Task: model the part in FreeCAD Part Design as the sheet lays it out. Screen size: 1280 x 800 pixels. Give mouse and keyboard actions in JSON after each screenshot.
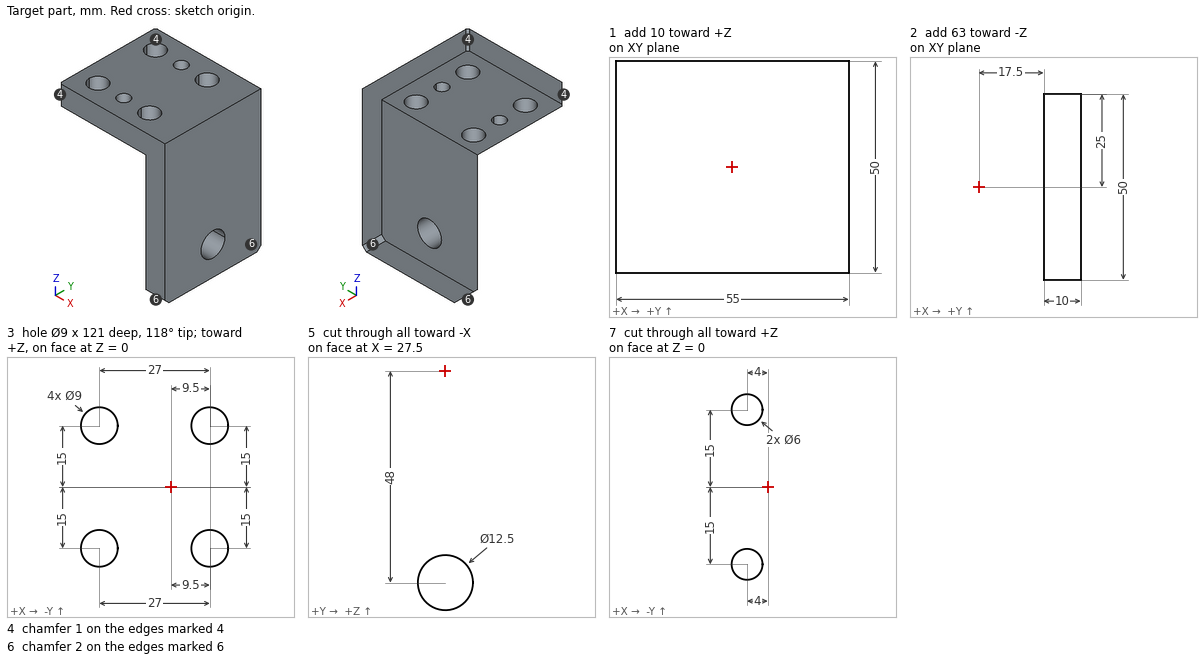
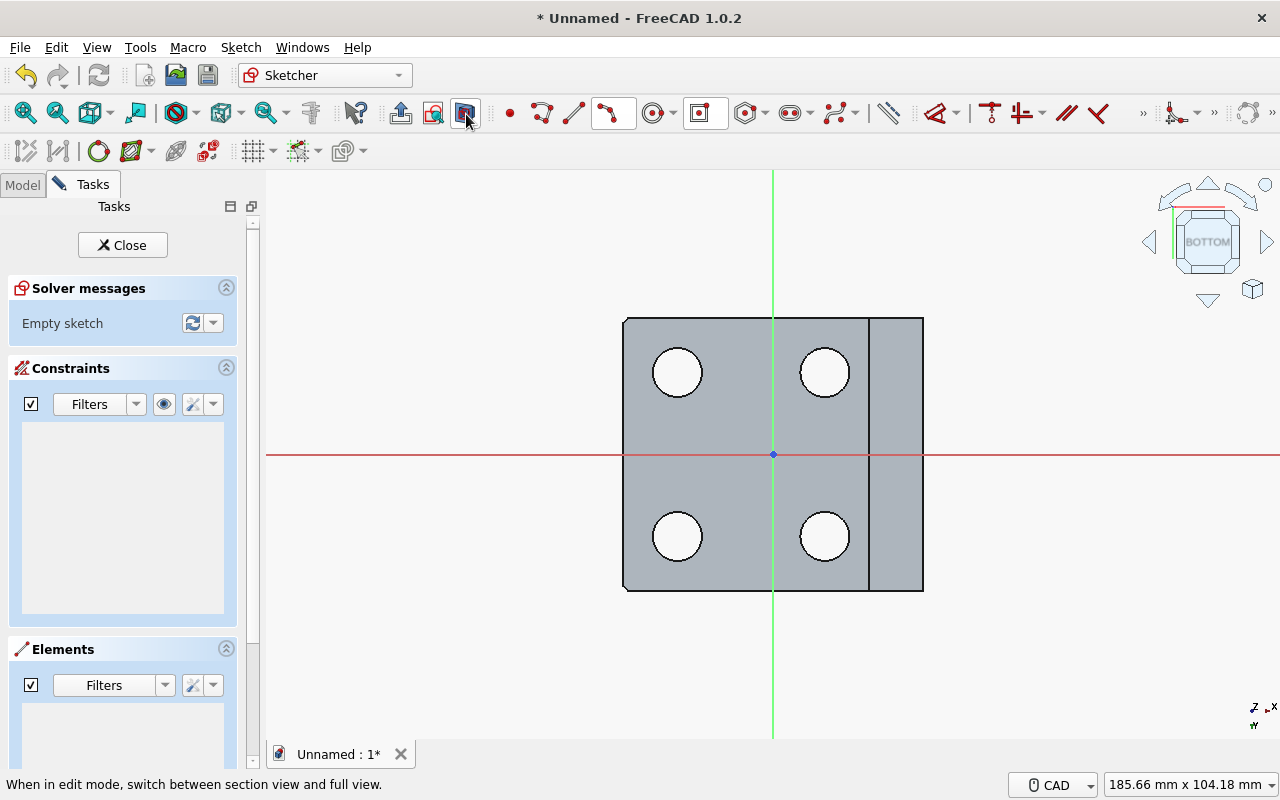
{"action": "scroll", "coordinate": [814, 455], "scroll_direction": "up", "scroll_amount": 3}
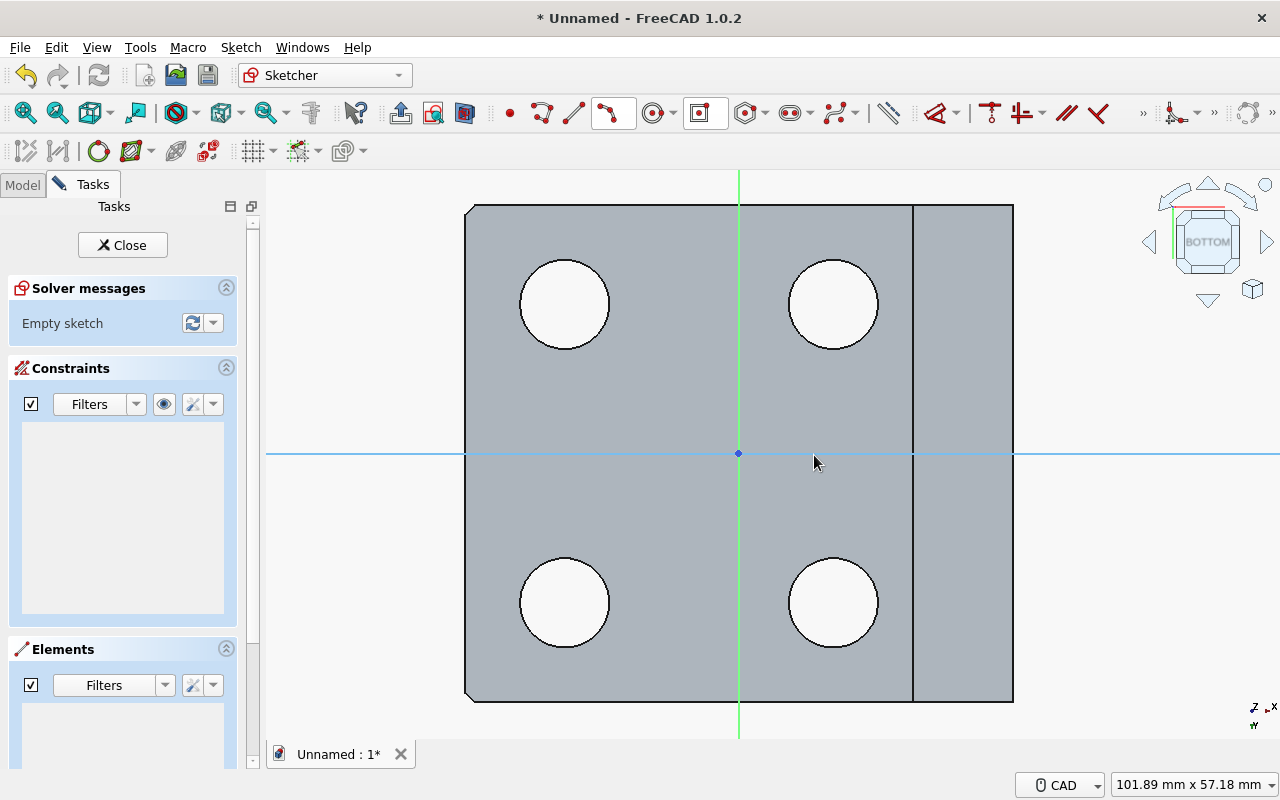
{"action": "left_click", "coordinate": [654, 114]}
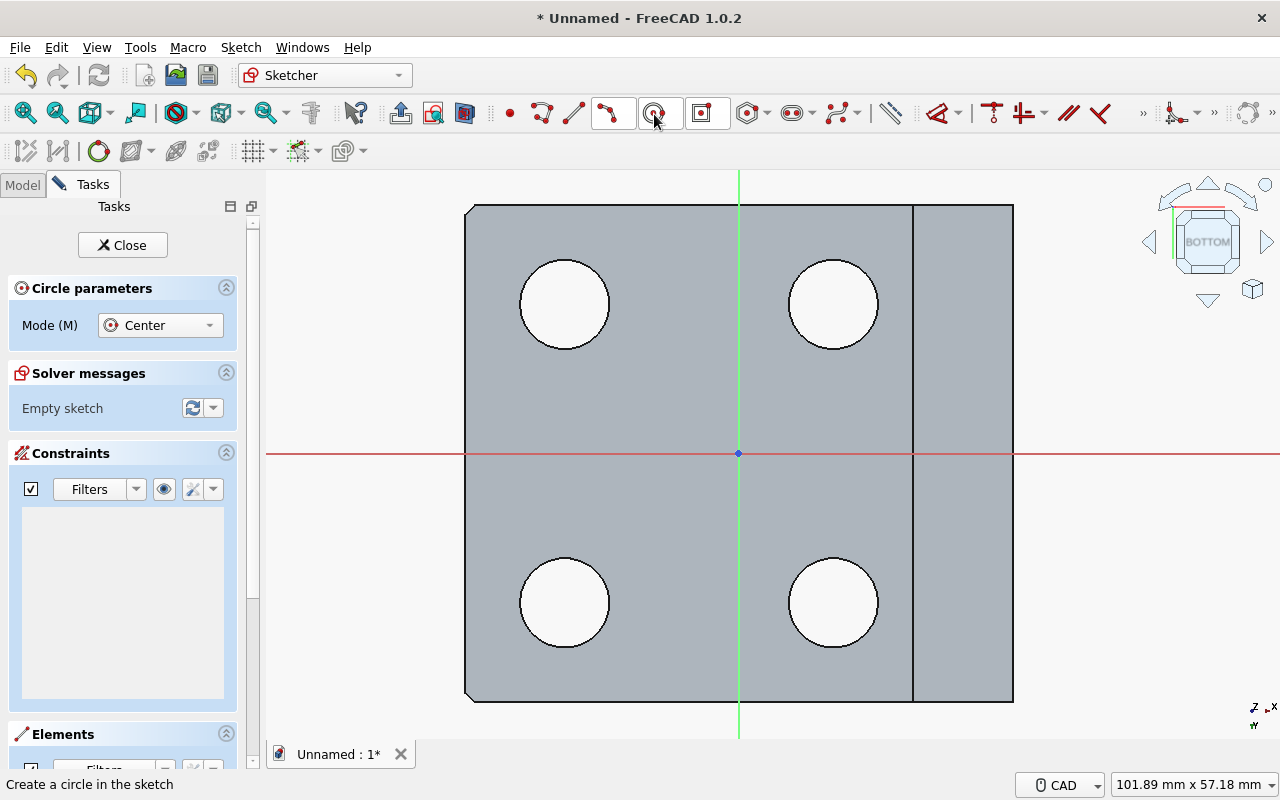
{"action": "left_click", "coordinate": [699, 304]}
{"action": "left_click", "coordinate": [720, 283]}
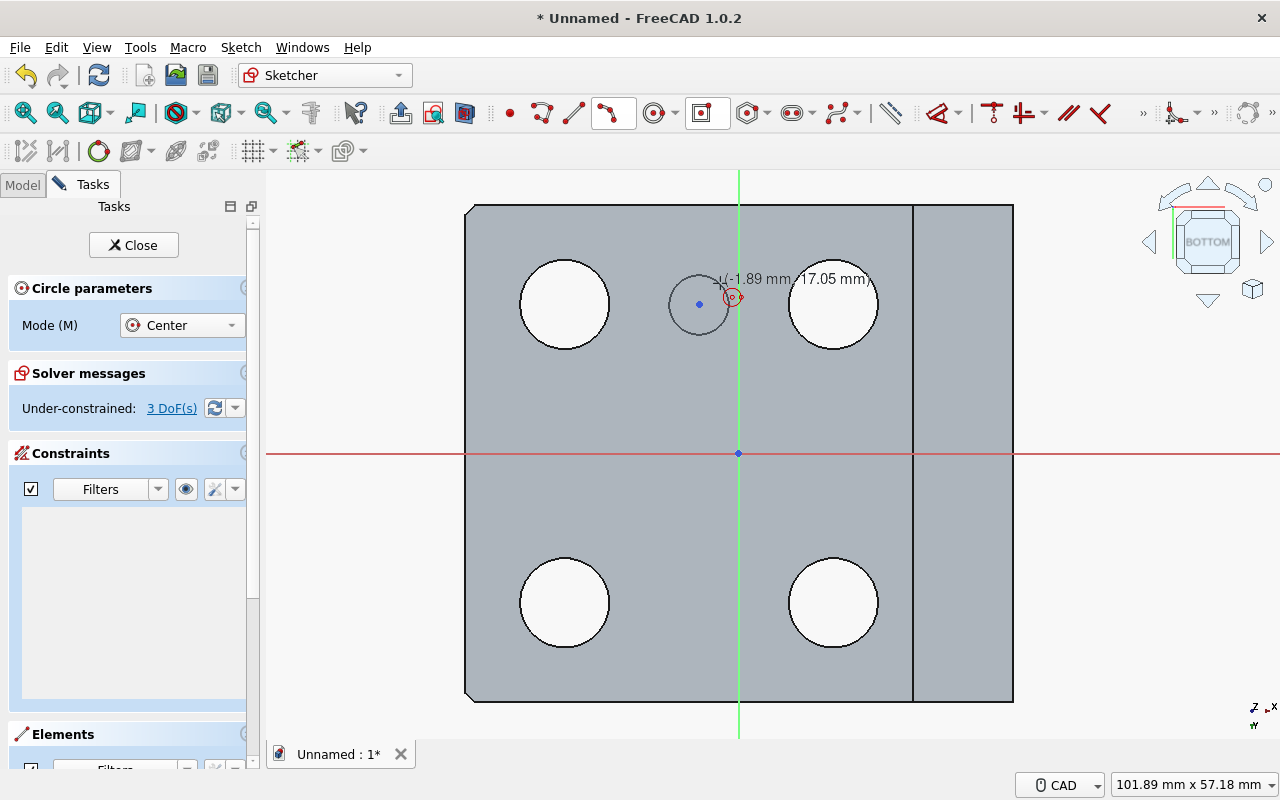
{"action": "left_click", "coordinate": [699, 603]}
{"action": "left_click", "coordinate": [720, 582]}
{"action": "key", "text": "Escape"}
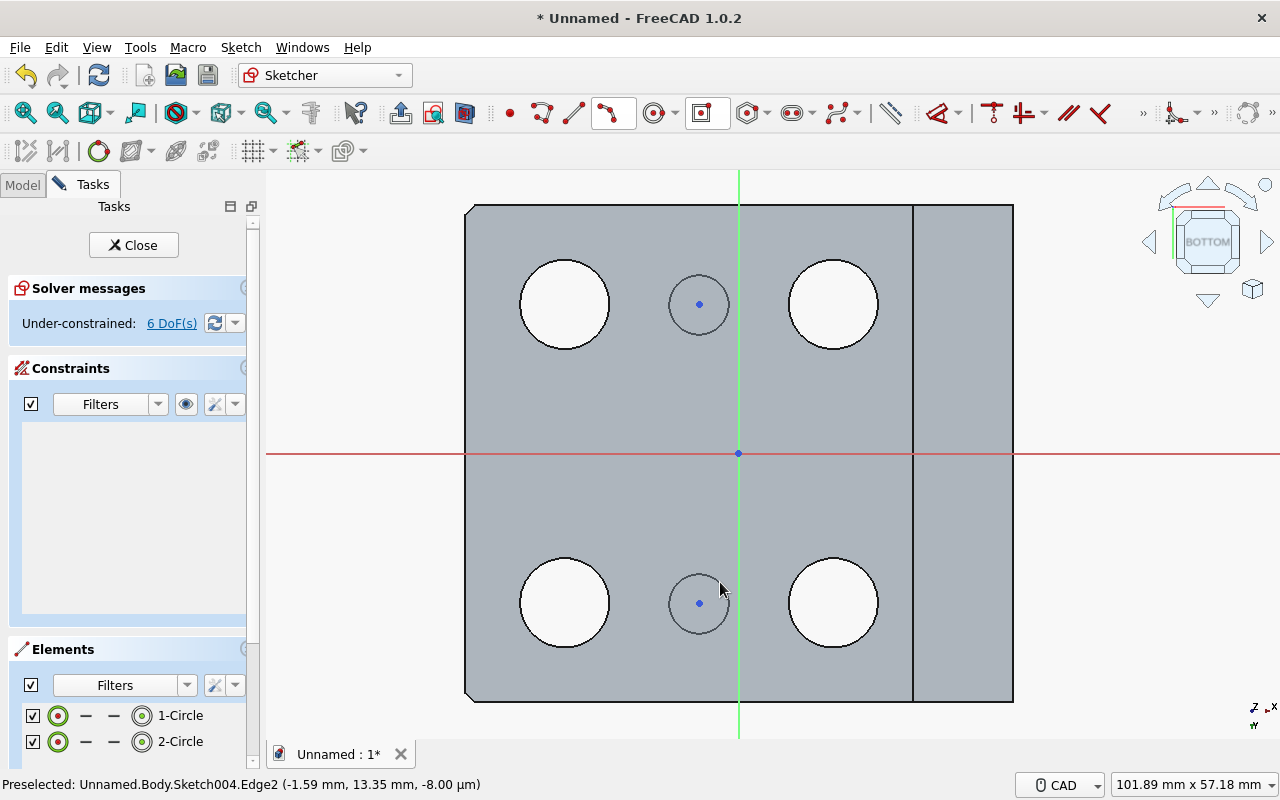
{"action": "left_click", "coordinate": [720, 284]}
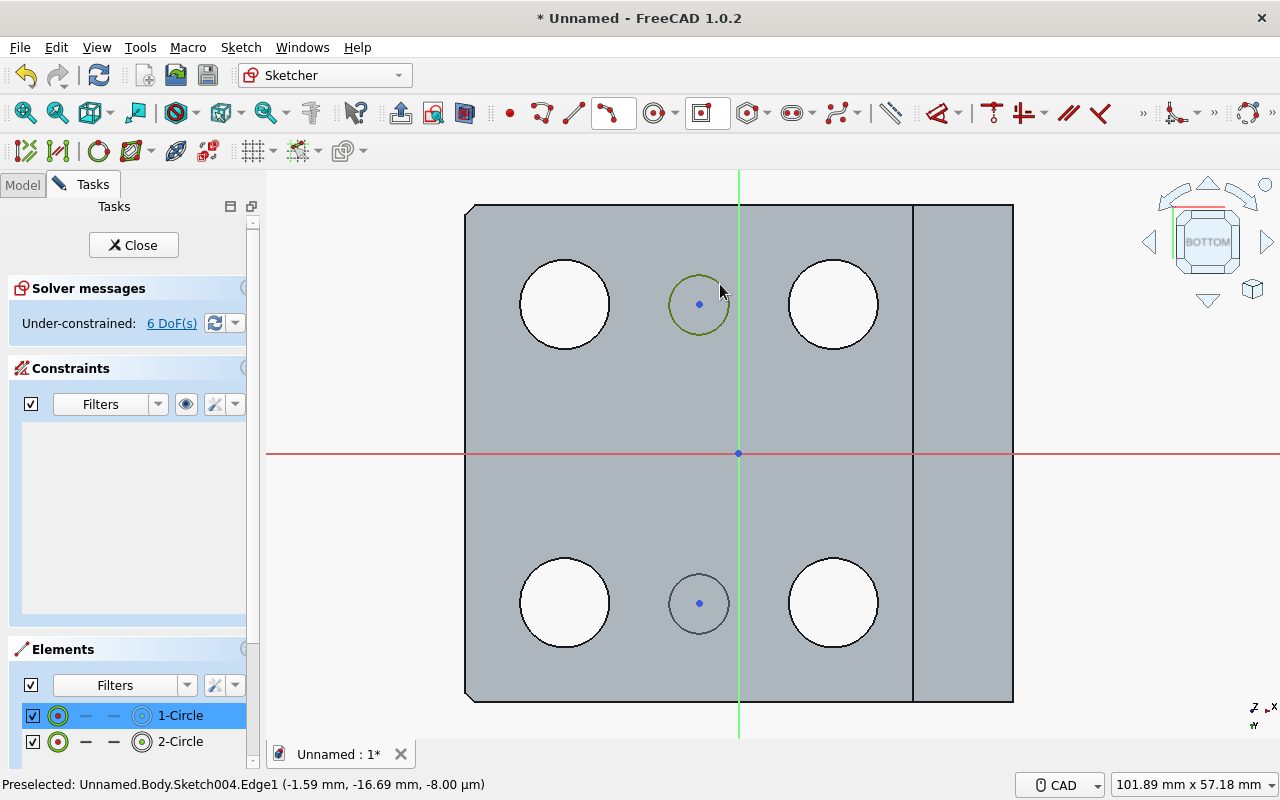
{"action": "left_click", "coordinate": [720, 583]}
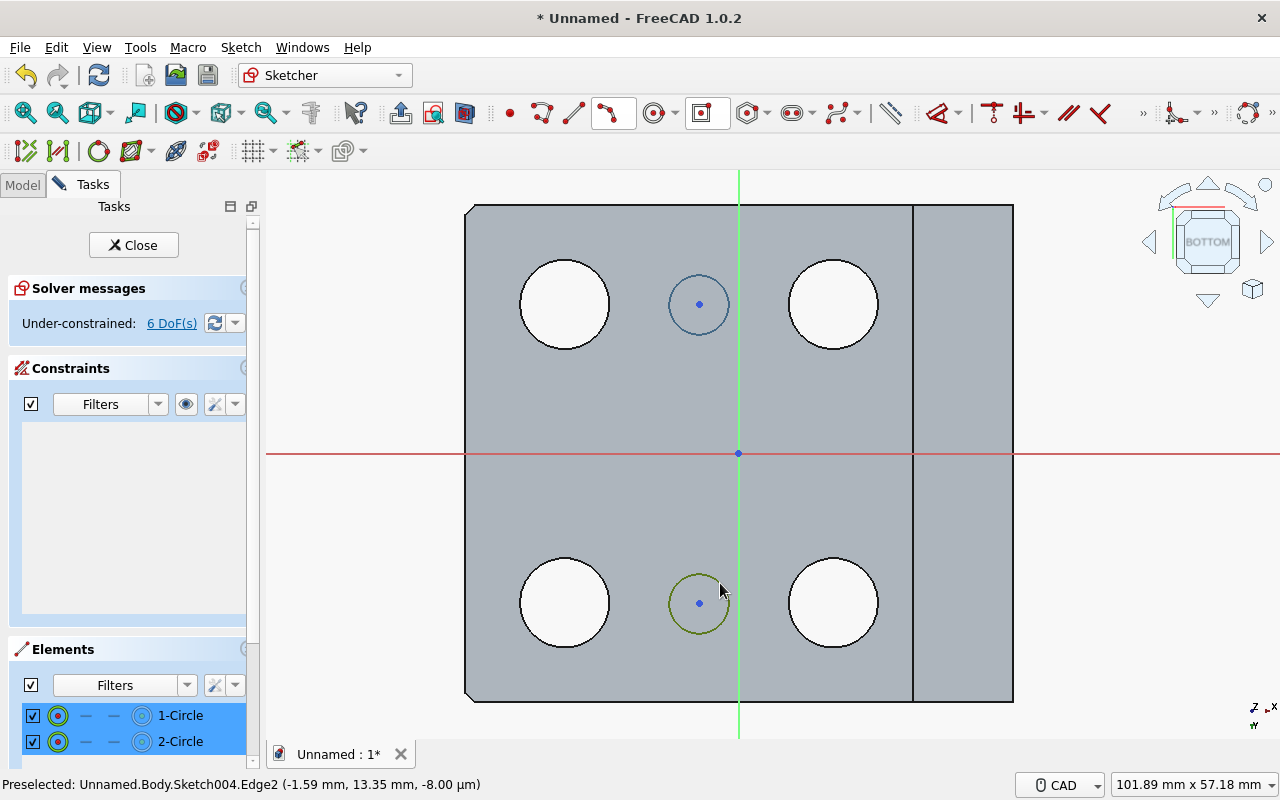
{"action": "key", "text": "e"}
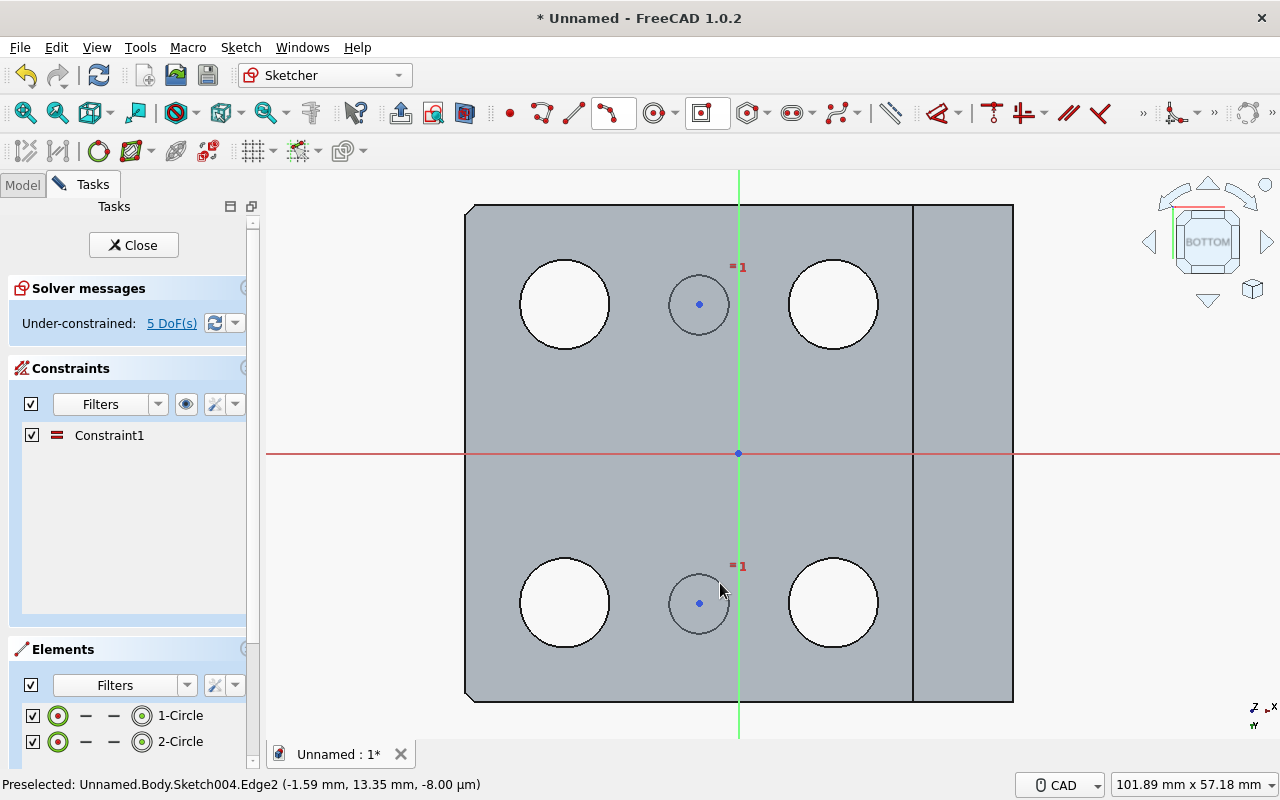
{"action": "left_click", "coordinate": [938, 114]}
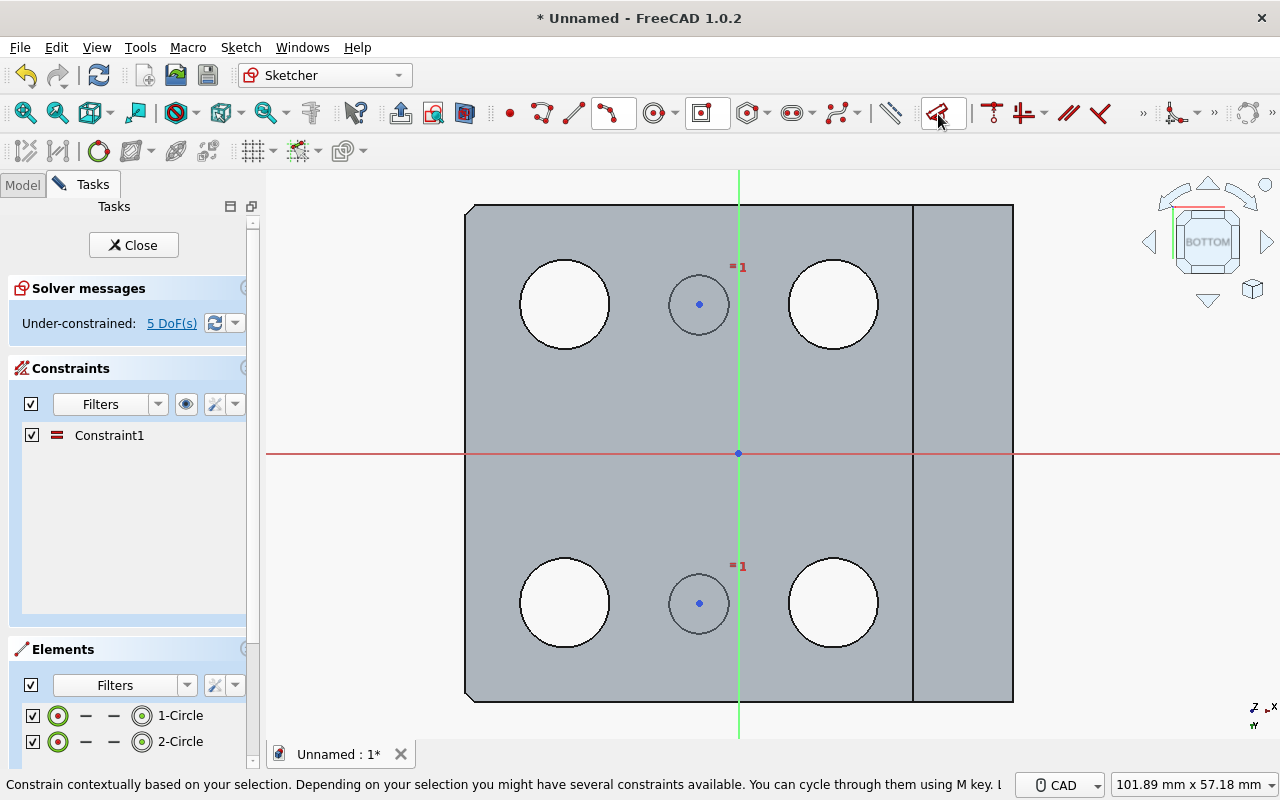
{"action": "left_click", "coordinate": [720, 284]}
{"action": "left_click", "coordinate": [758, 288]}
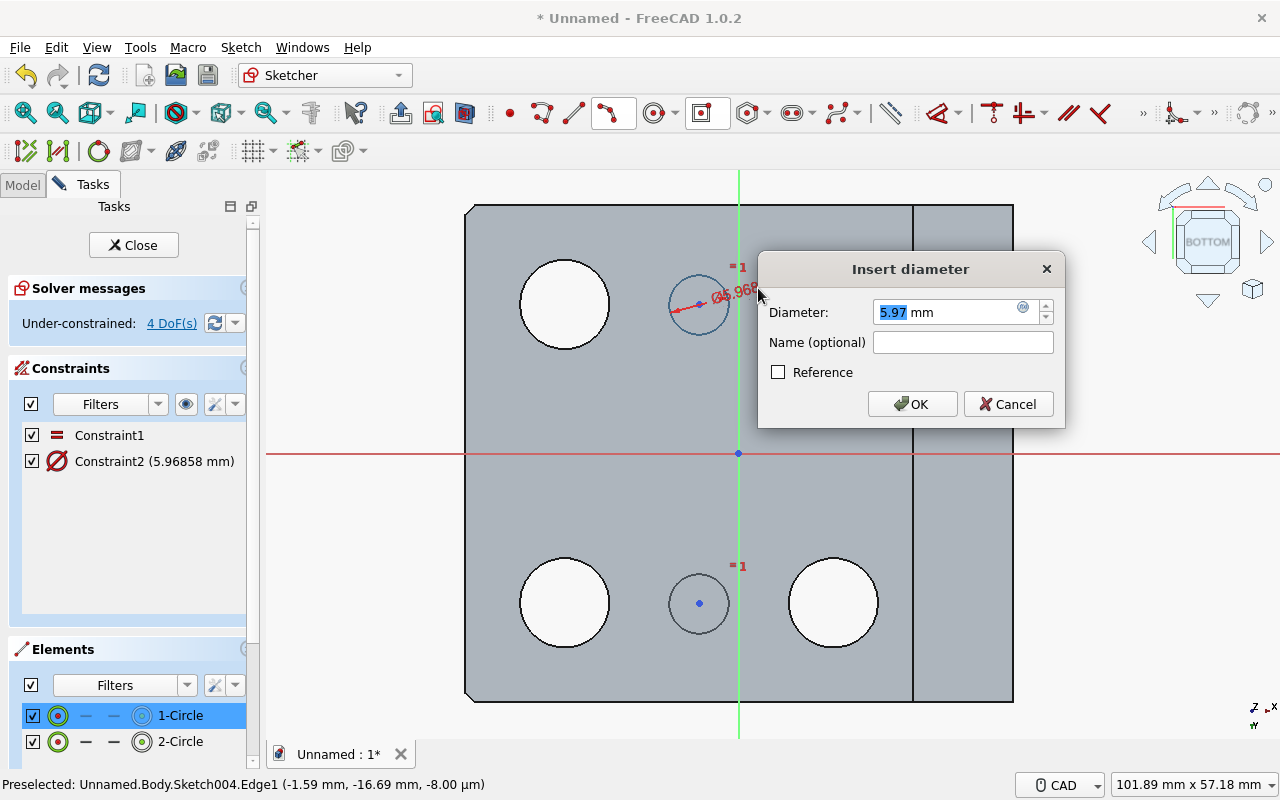
{"action": "type", "text": "6"}
{"action": "key", "text": "Return"}